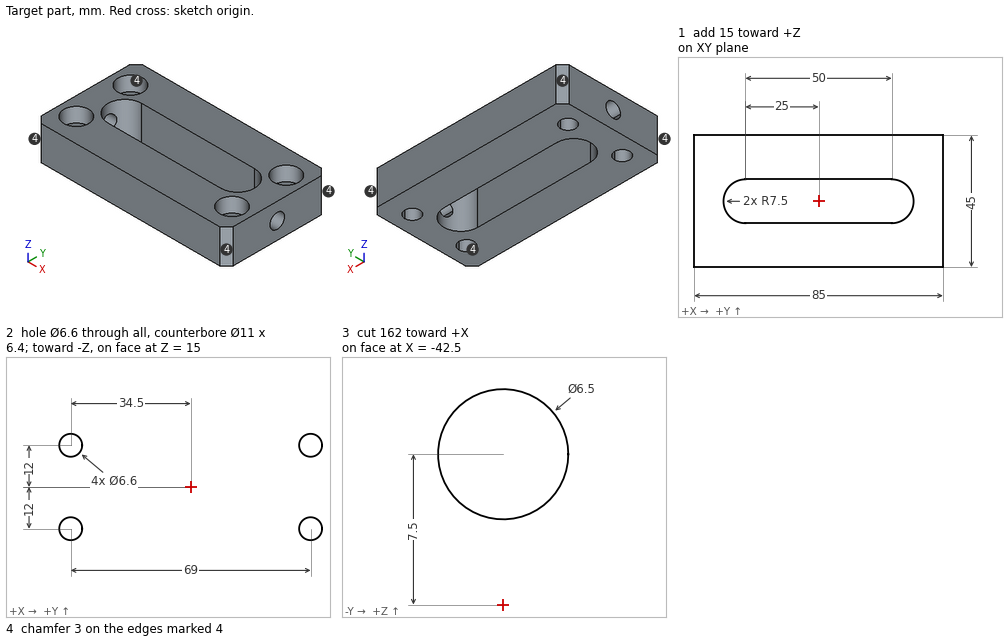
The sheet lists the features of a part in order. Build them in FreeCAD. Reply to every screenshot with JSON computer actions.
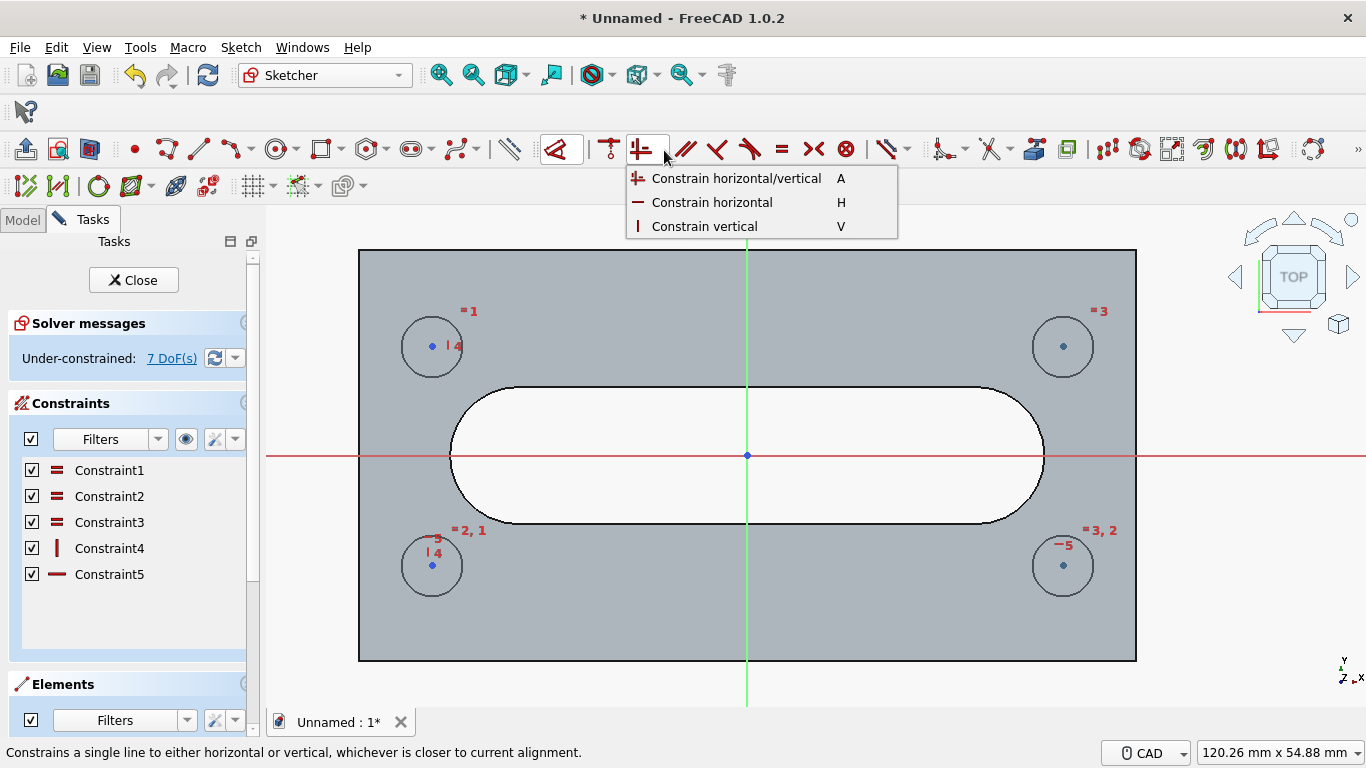
{"action": "left_click", "coordinate": [762, 226]}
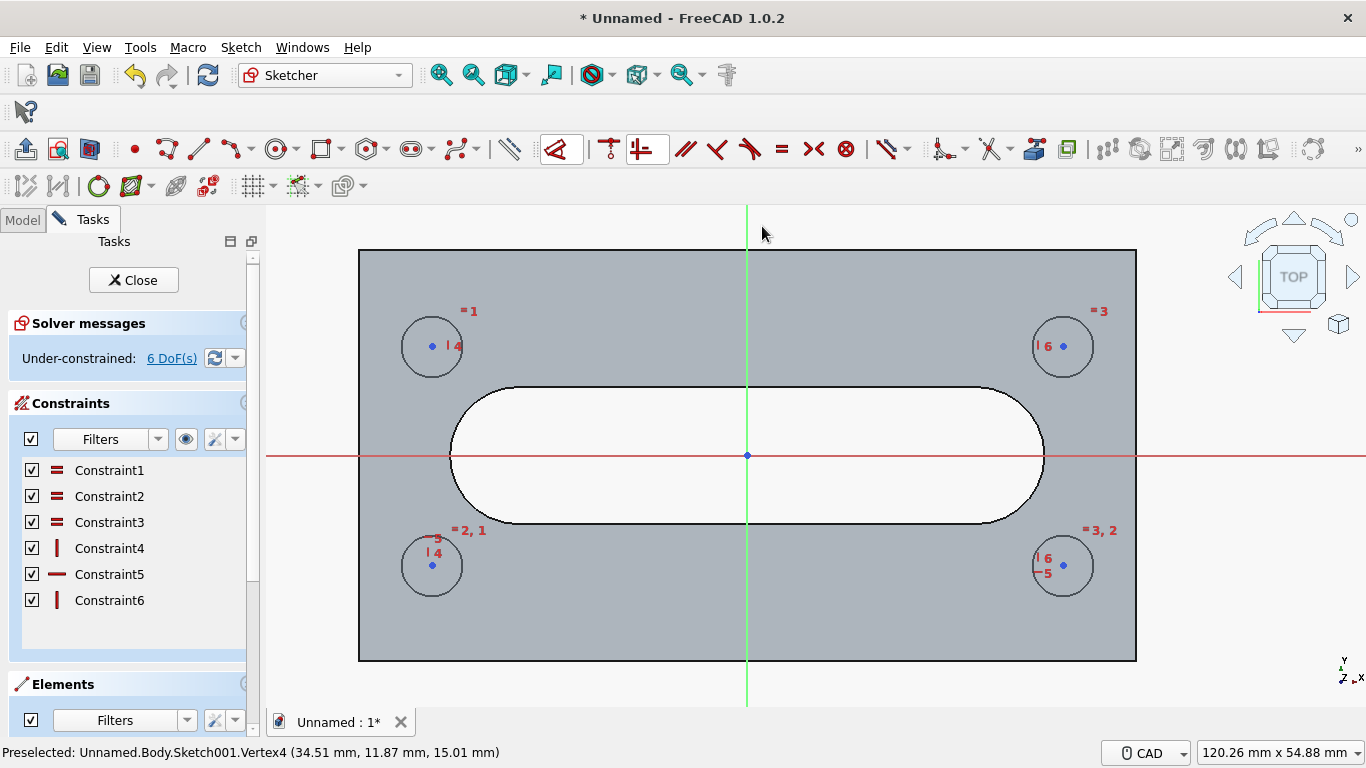
{"action": "left_click", "coordinate": [432, 347]}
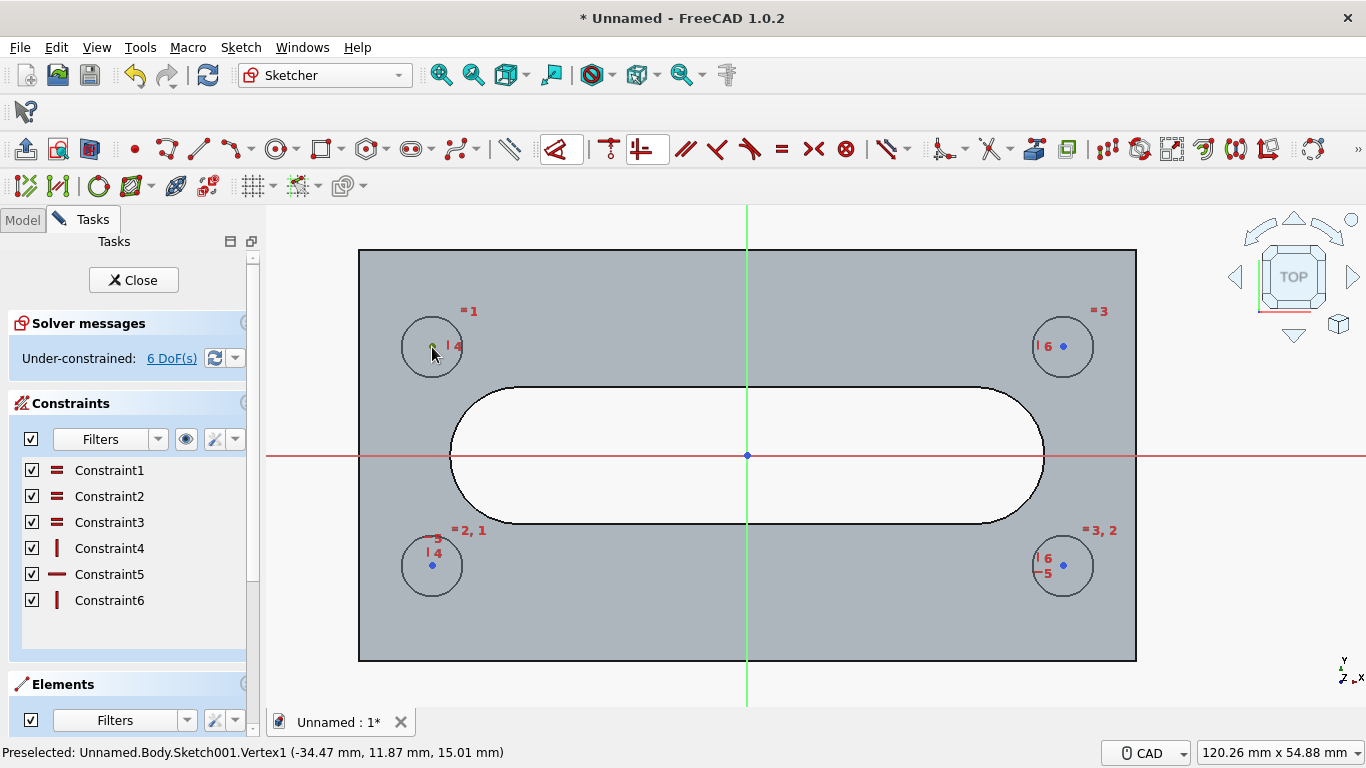
{"action": "left_click", "coordinate": [1063, 347]}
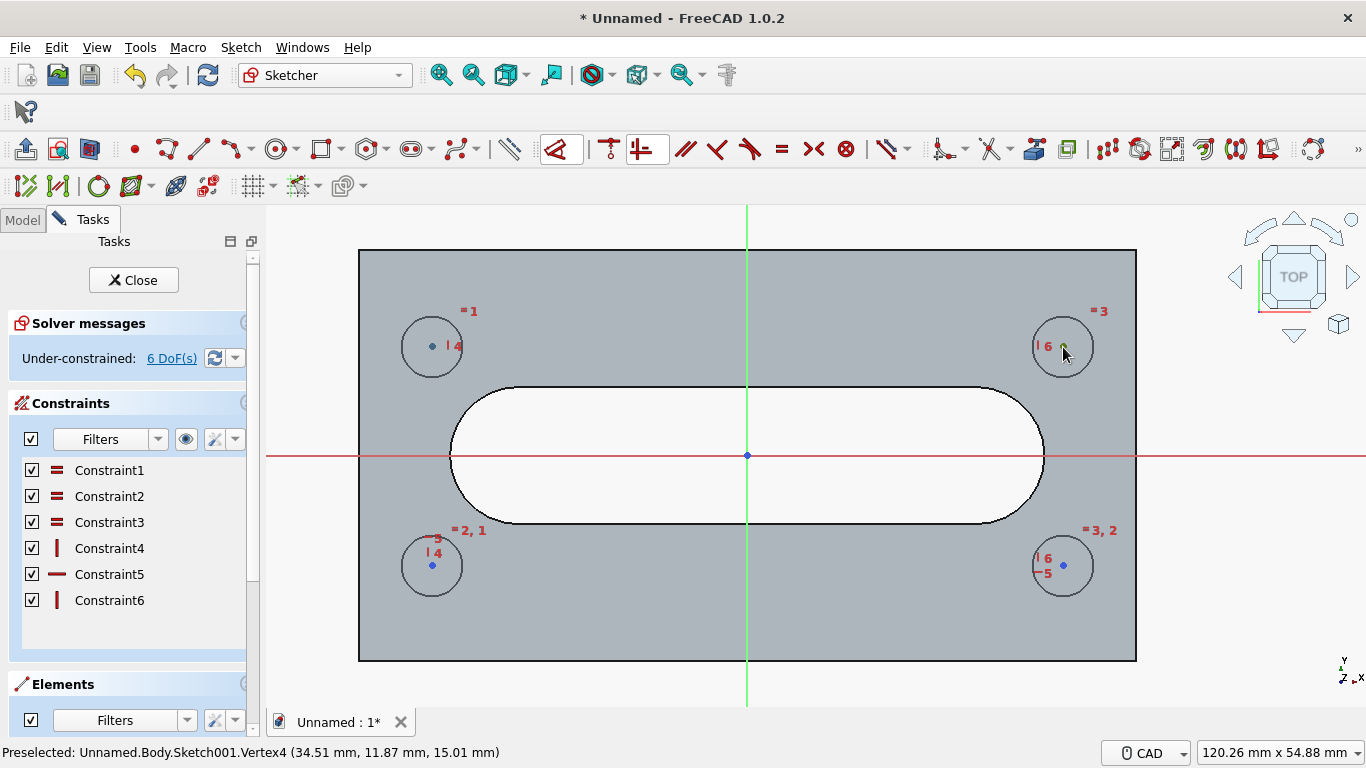
{"action": "left_click", "coordinate": [664, 150]}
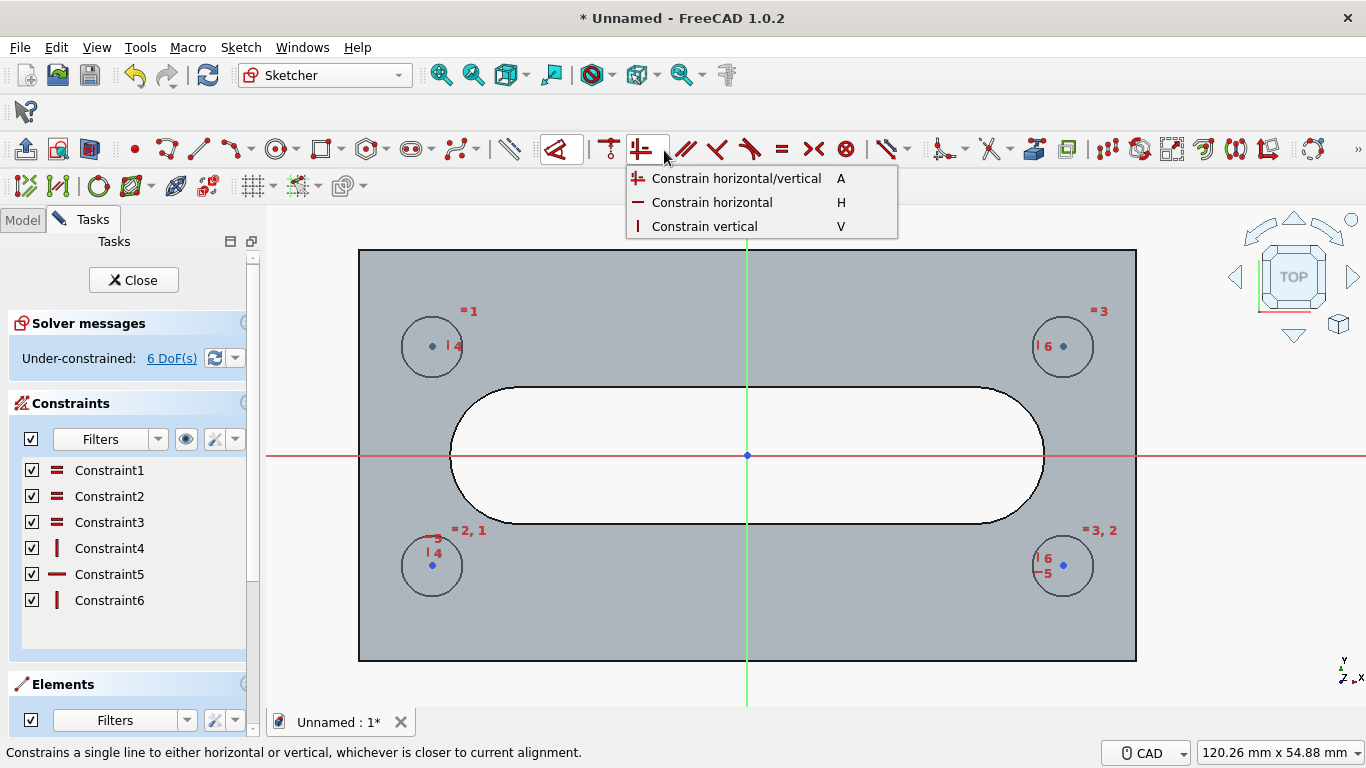
{"action": "left_click", "coordinate": [762, 202]}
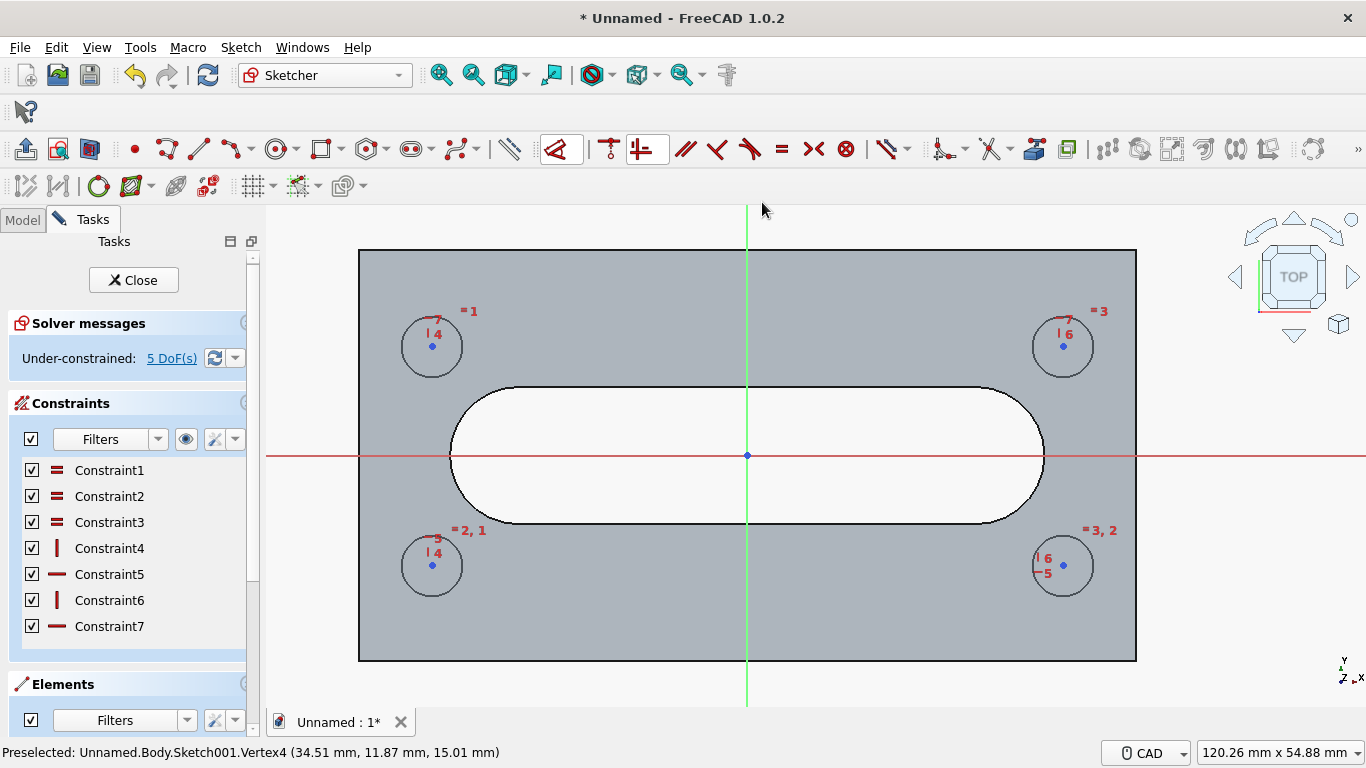
{"action": "left_click", "coordinate": [556, 150]}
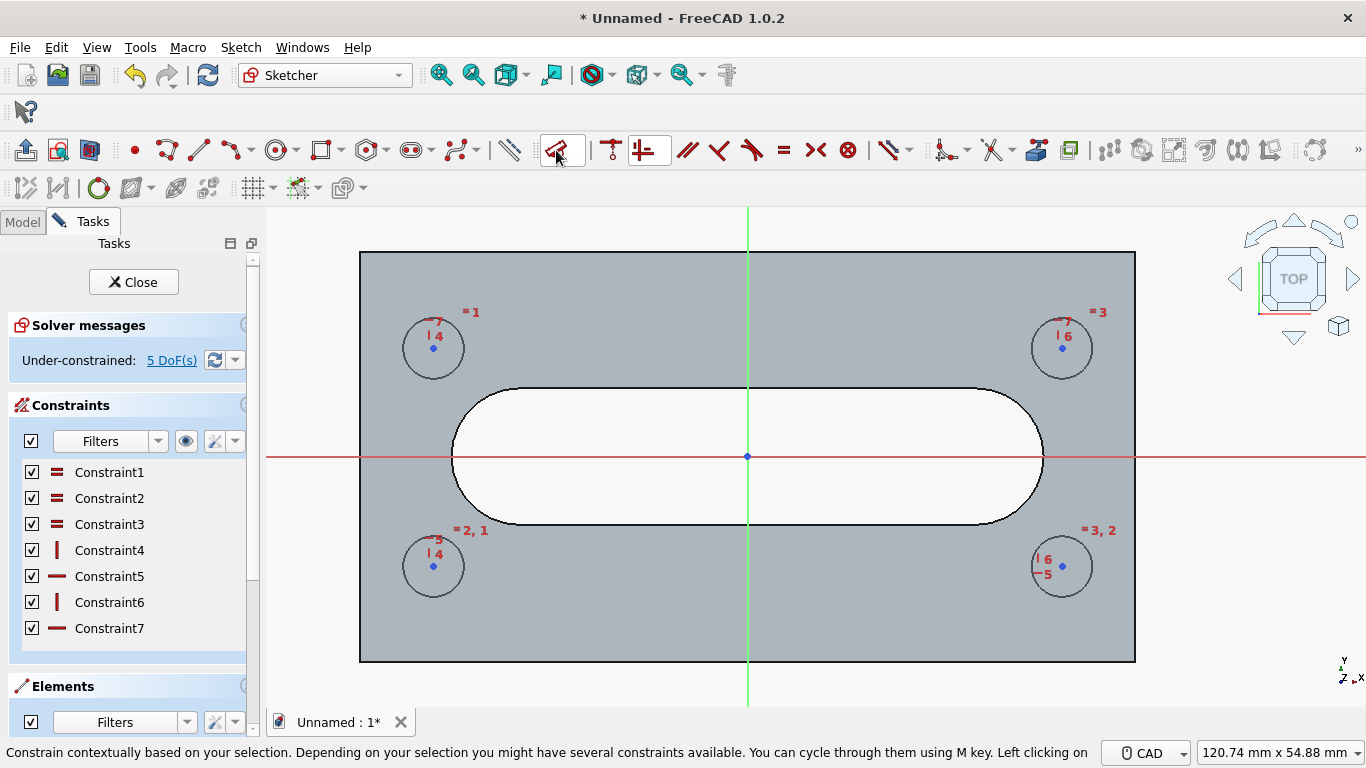
{"action": "left_click", "coordinate": [455, 327]}
{"action": "left_click", "coordinate": [478, 304]}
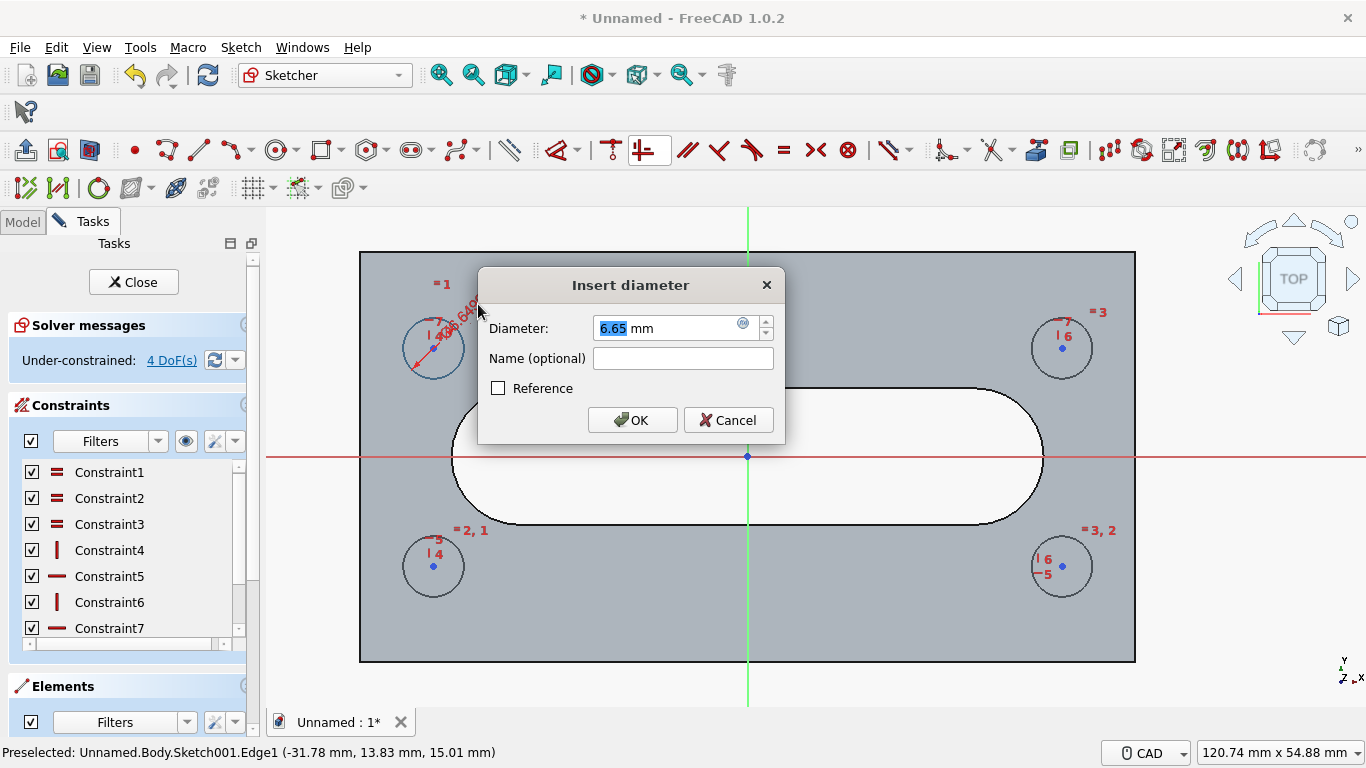
{"action": "type", "text": "6.6"}
{"action": "key", "text": "Return"}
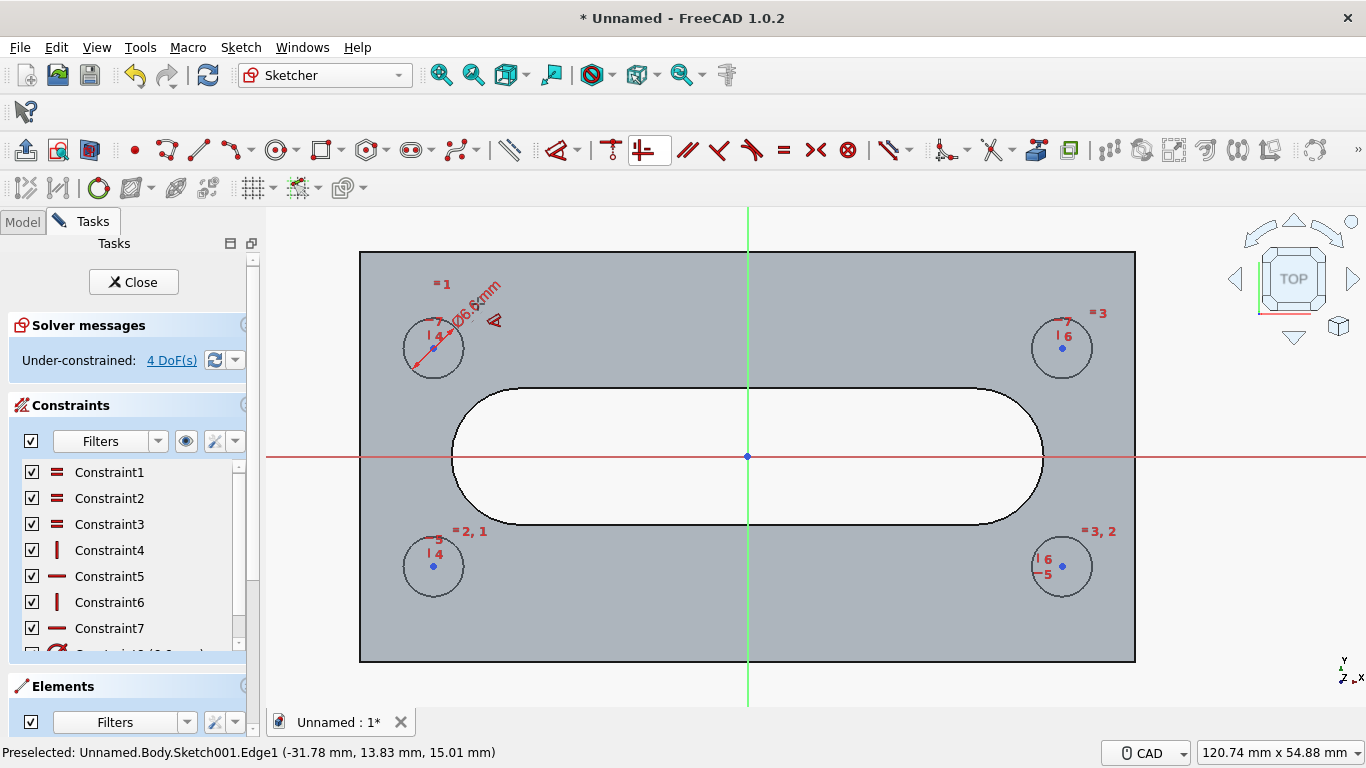
{"action": "left_click", "coordinate": [434, 348]}
{"action": "left_click", "coordinate": [400, 403]}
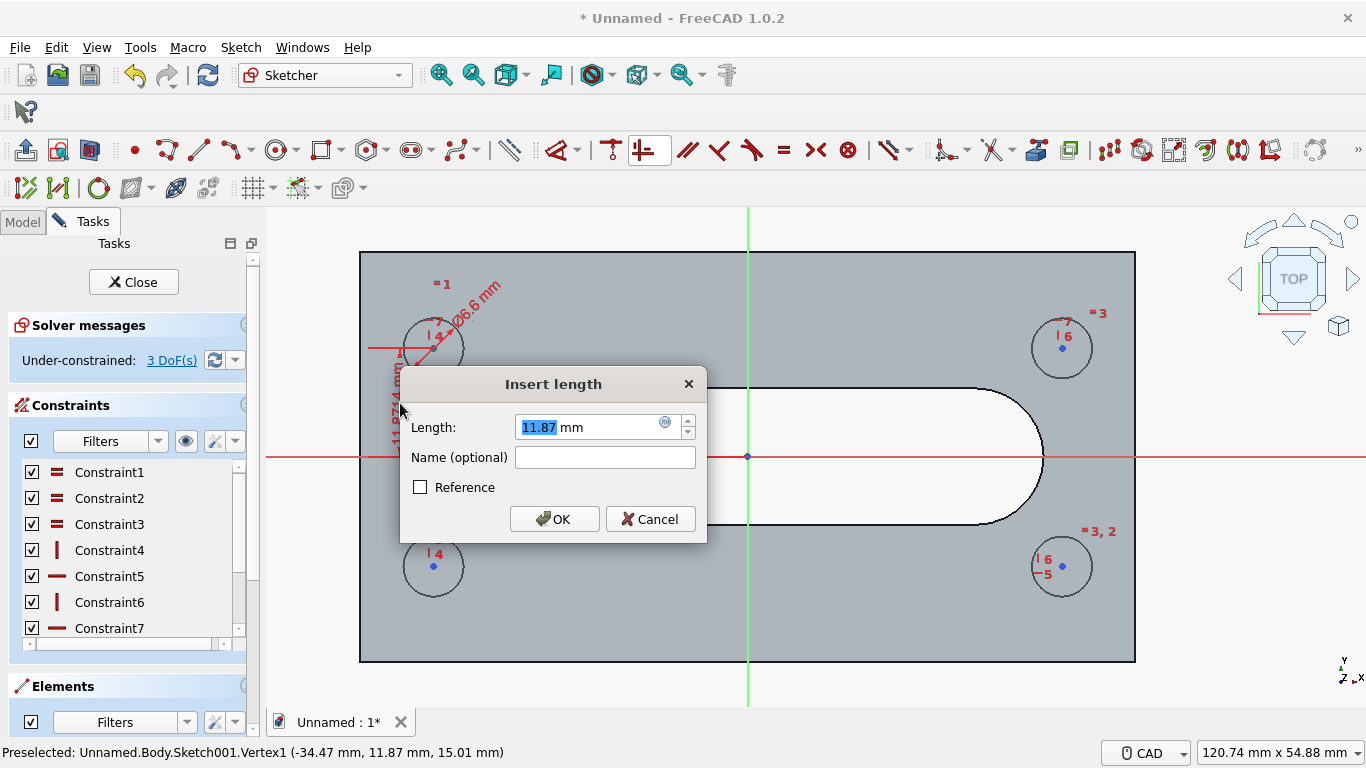
{"action": "type", "text": "12"}
{"action": "key", "text": "Return"}